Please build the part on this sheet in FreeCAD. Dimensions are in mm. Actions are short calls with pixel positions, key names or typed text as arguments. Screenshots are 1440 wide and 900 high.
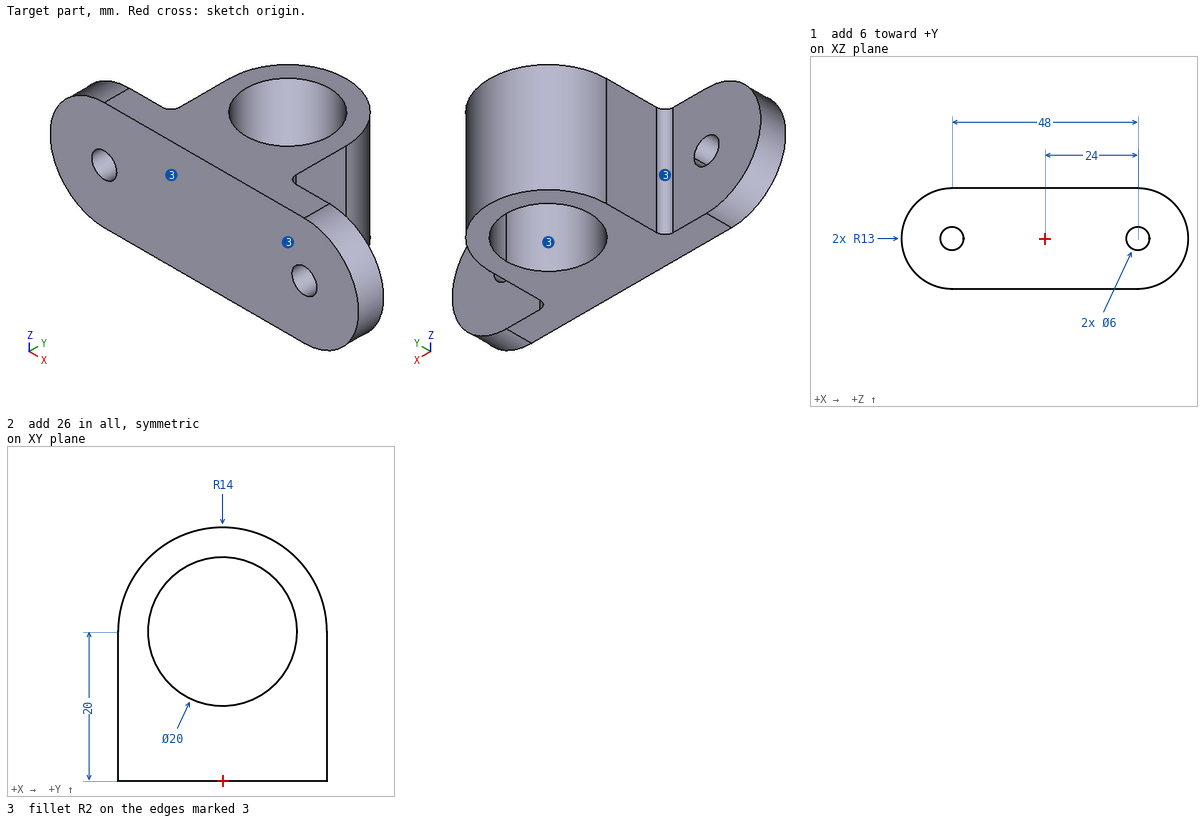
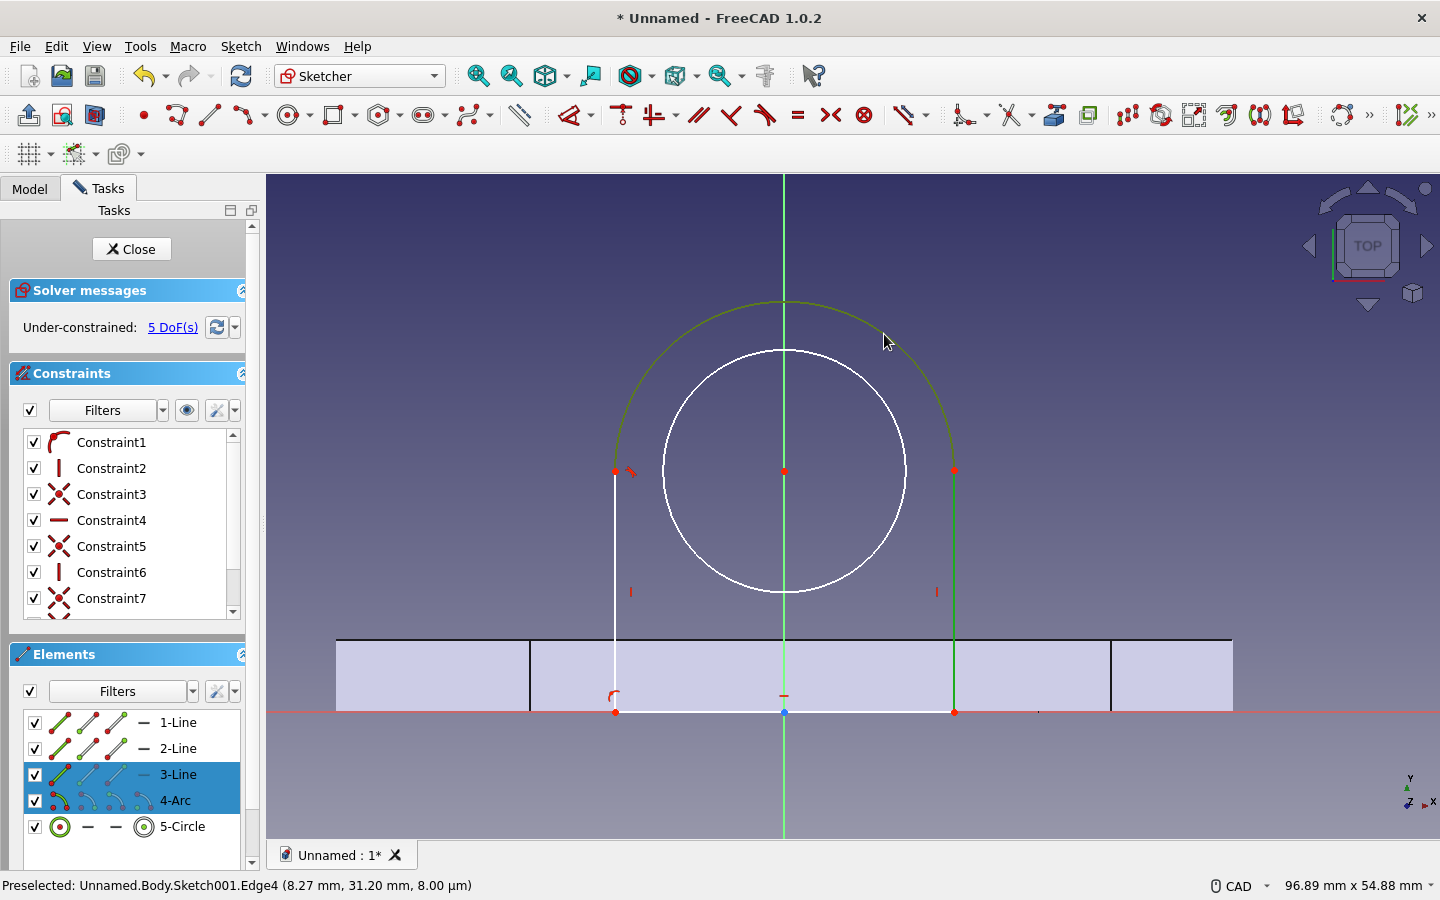
key(t)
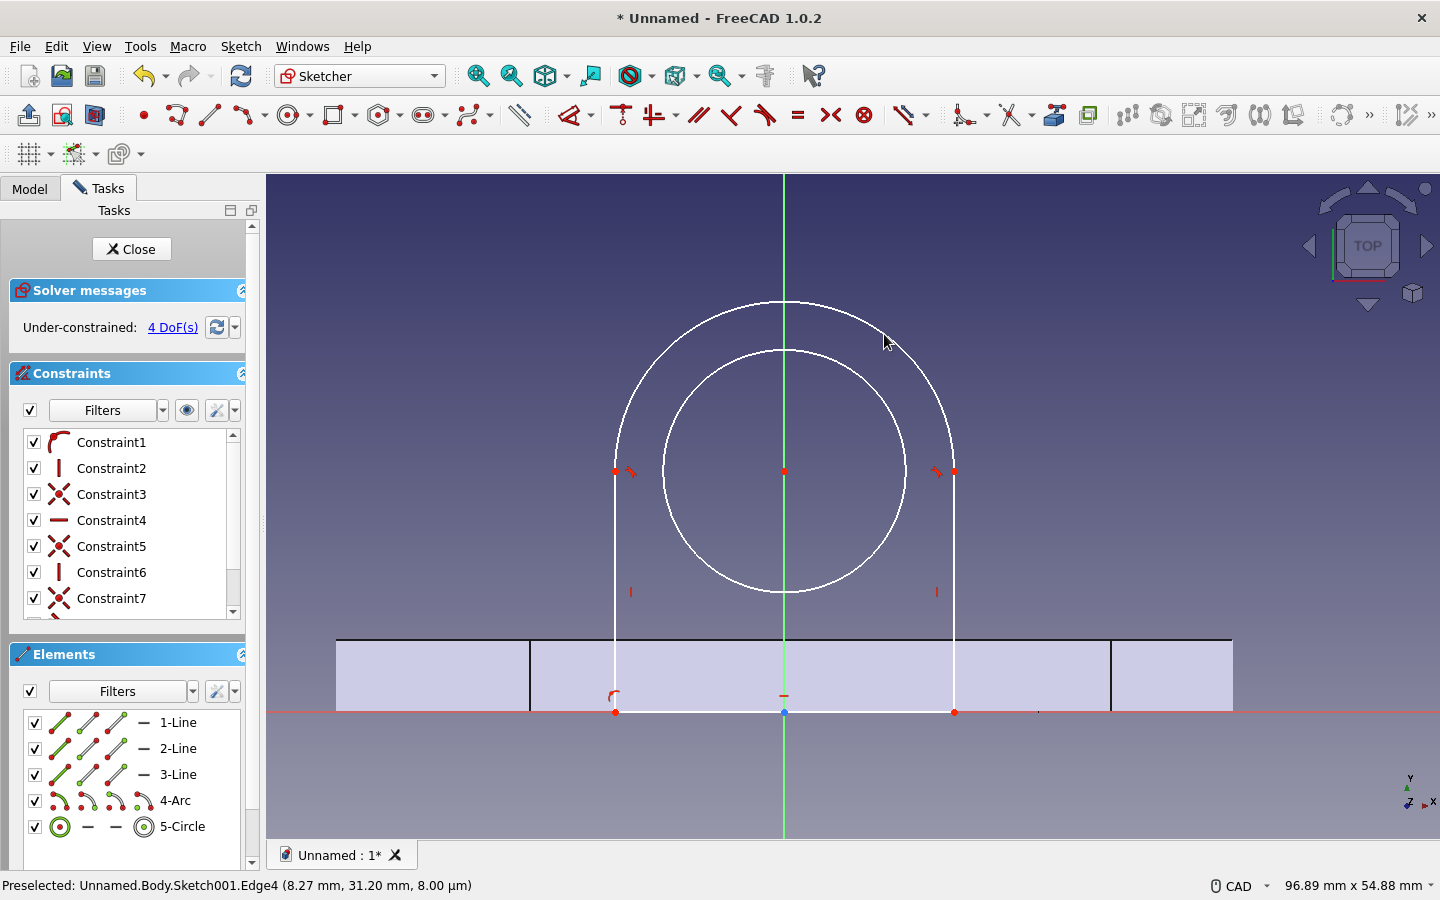
click(784, 471)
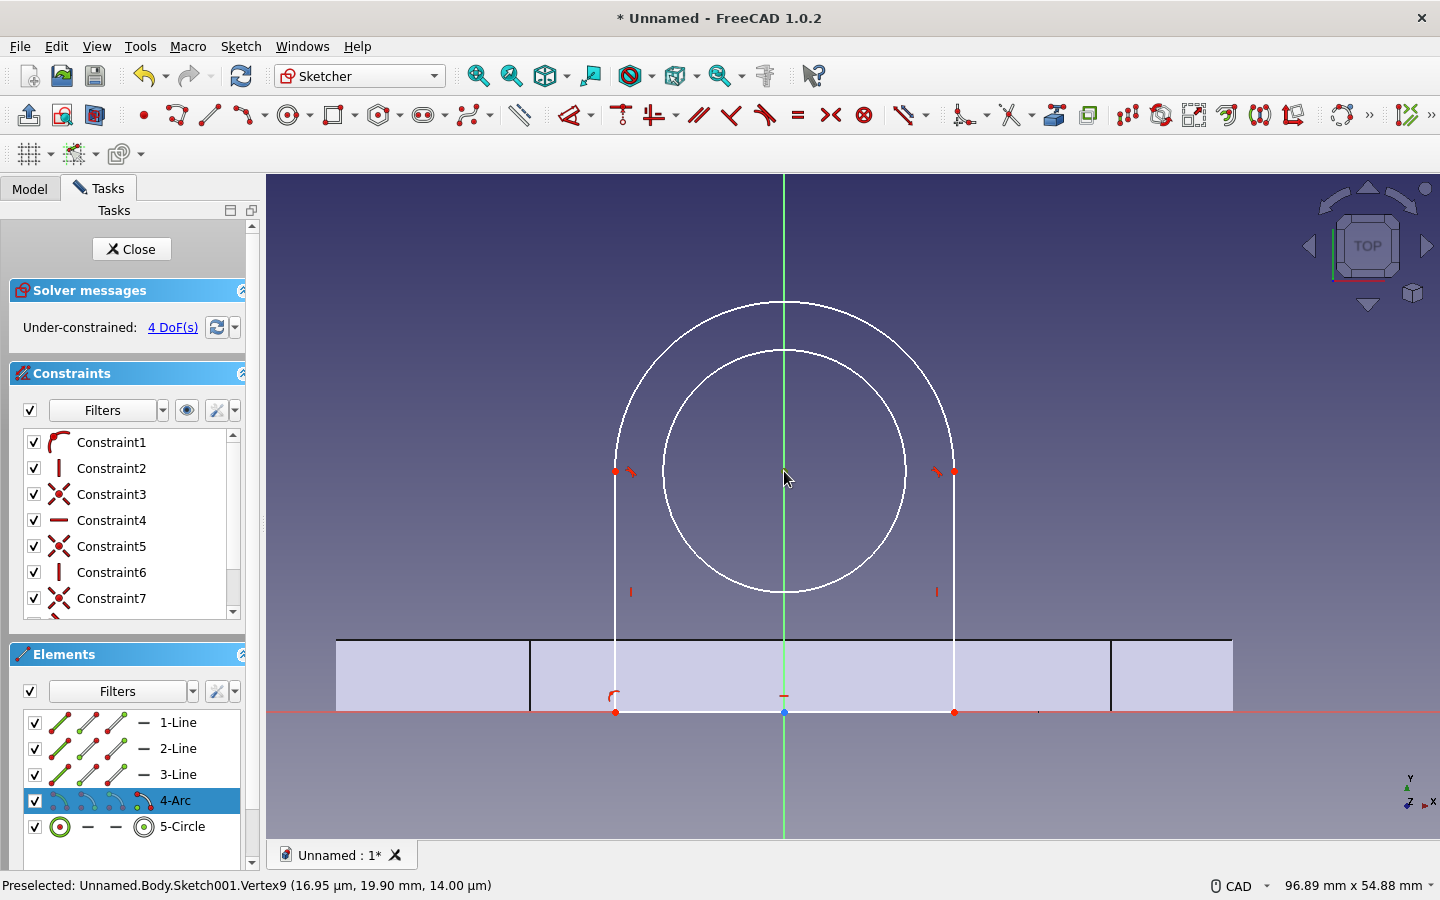
click(784, 768)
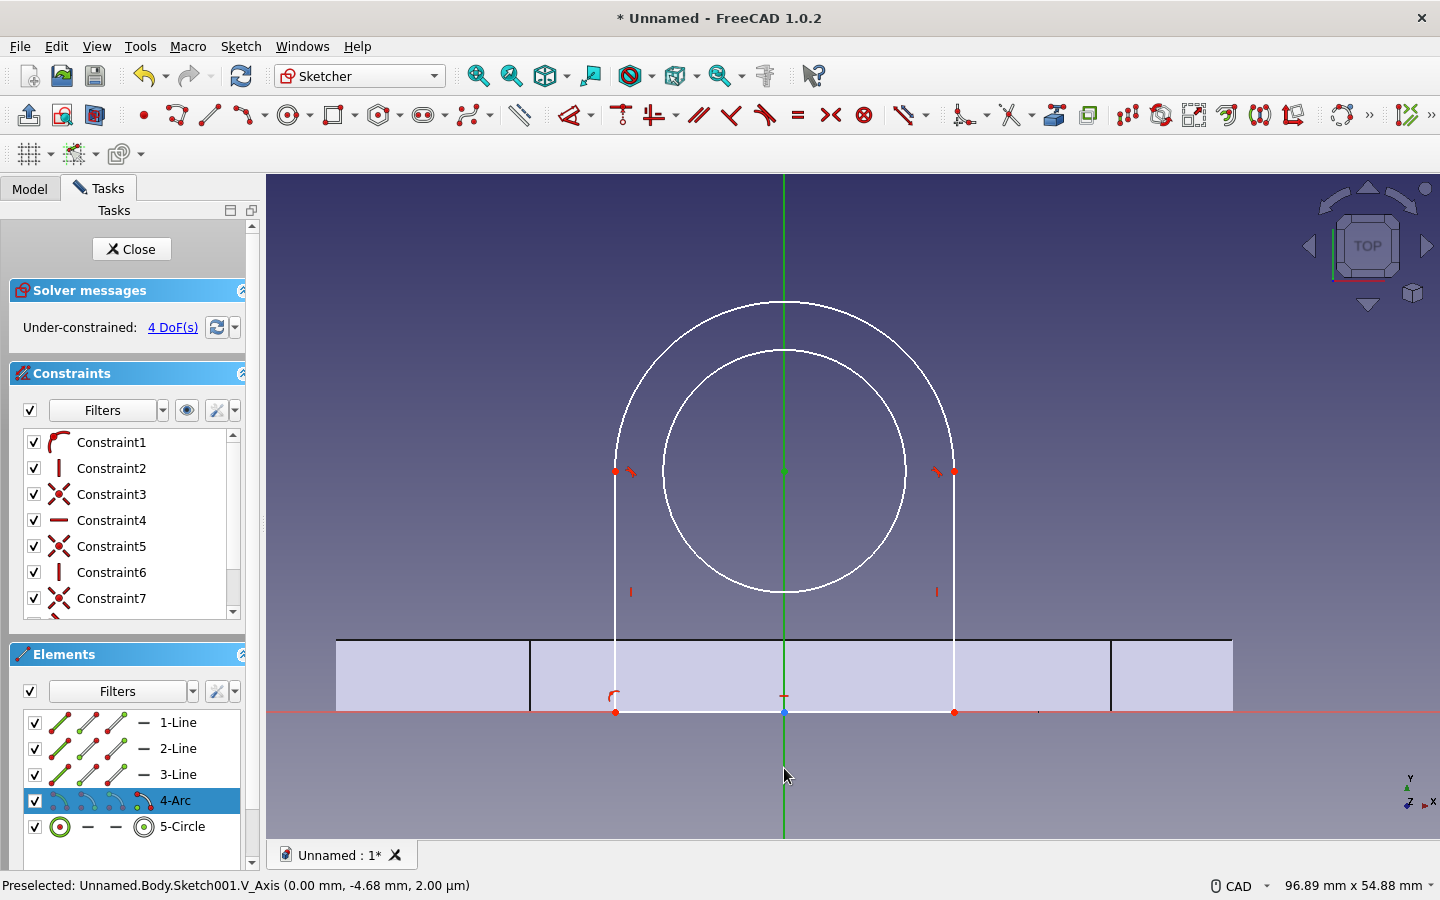
key(c)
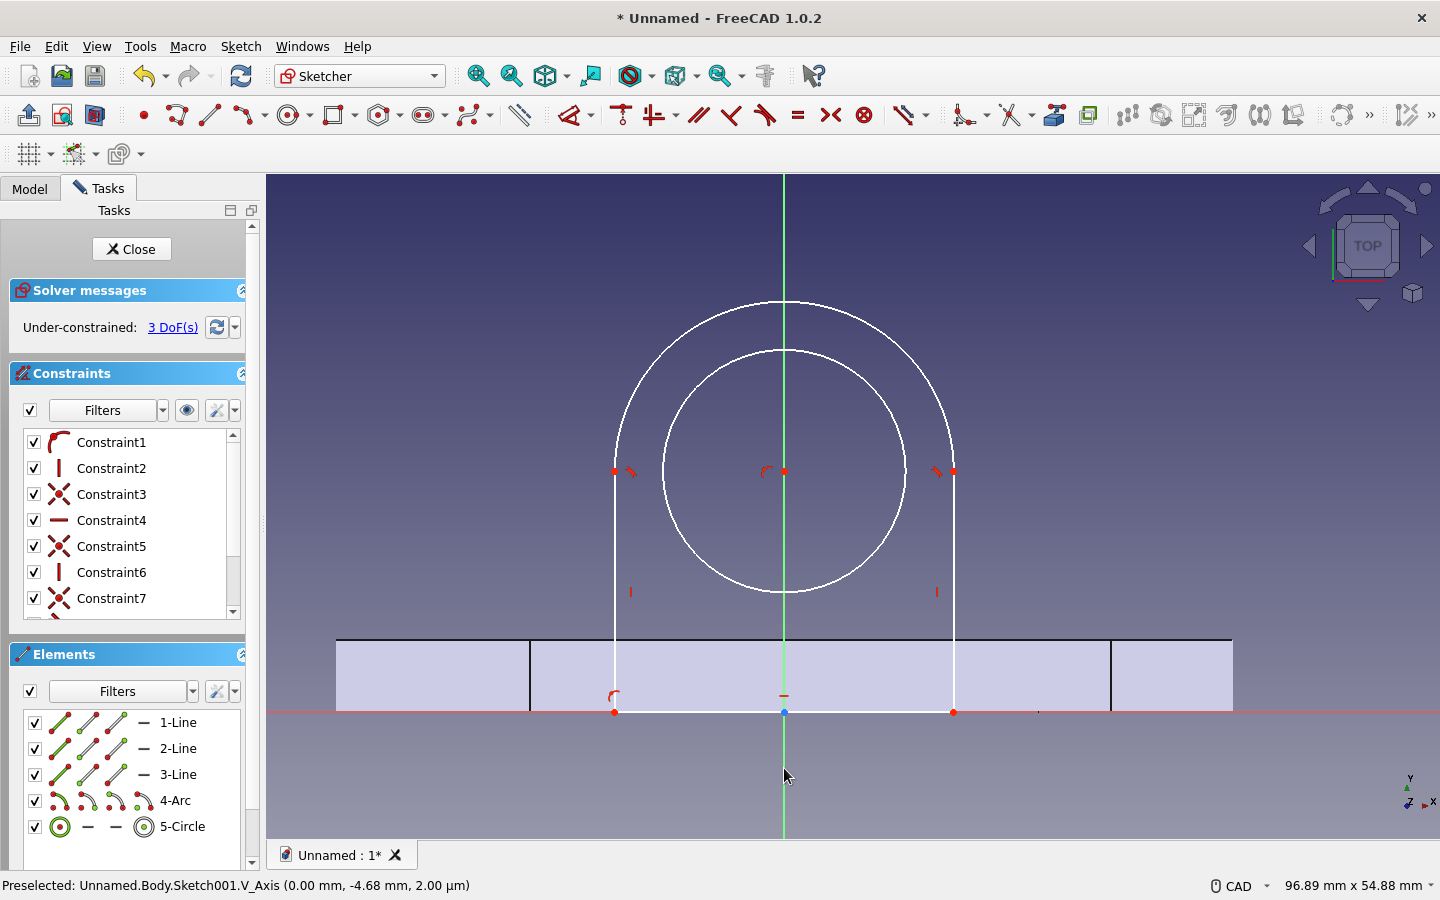
click(884, 334)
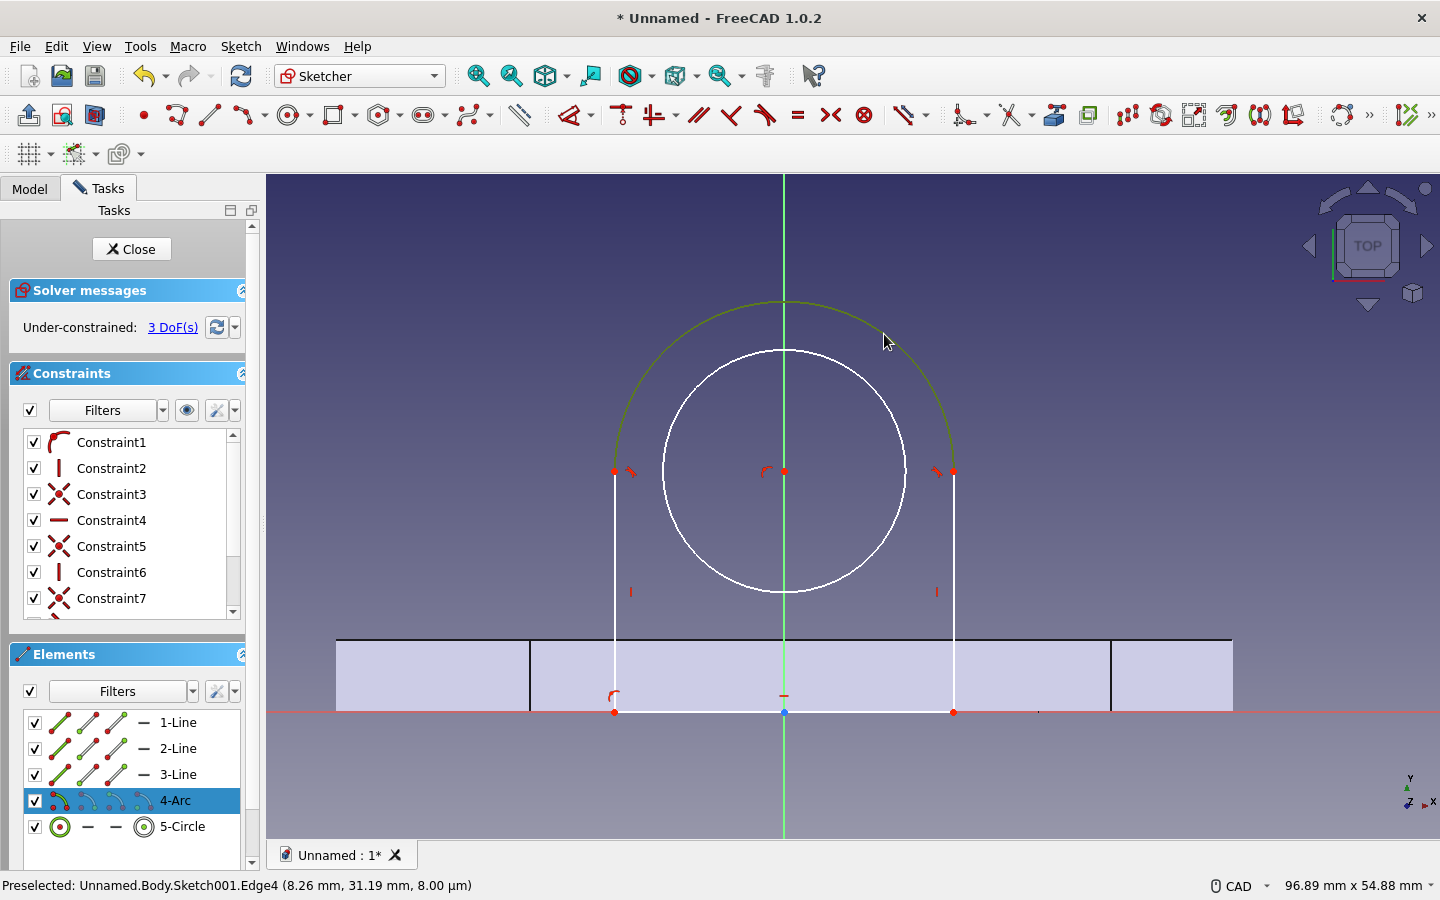
key(k)
key(r)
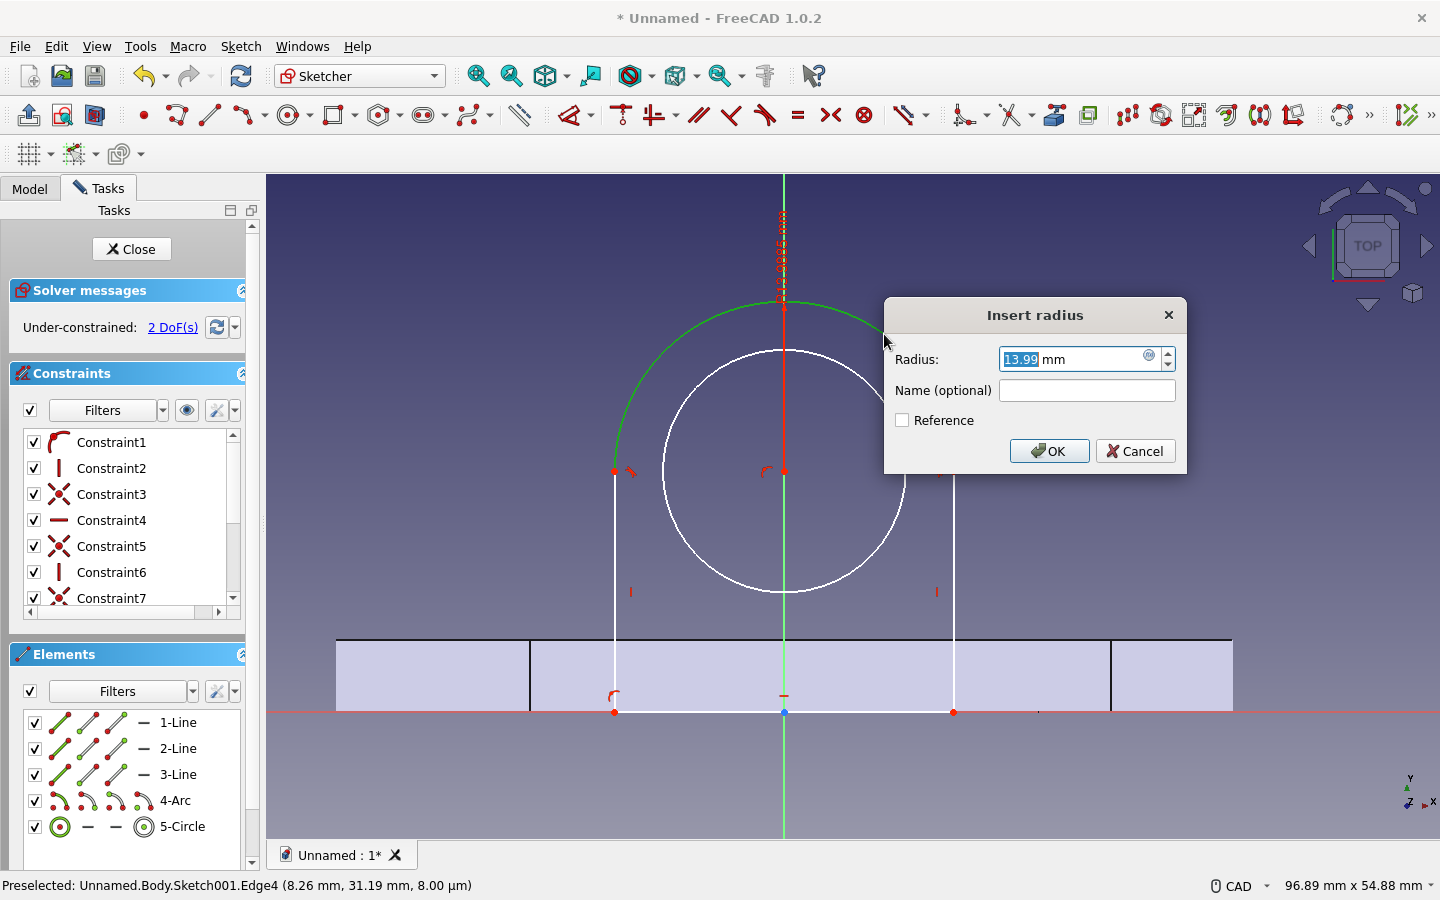
text(14)
key(Return)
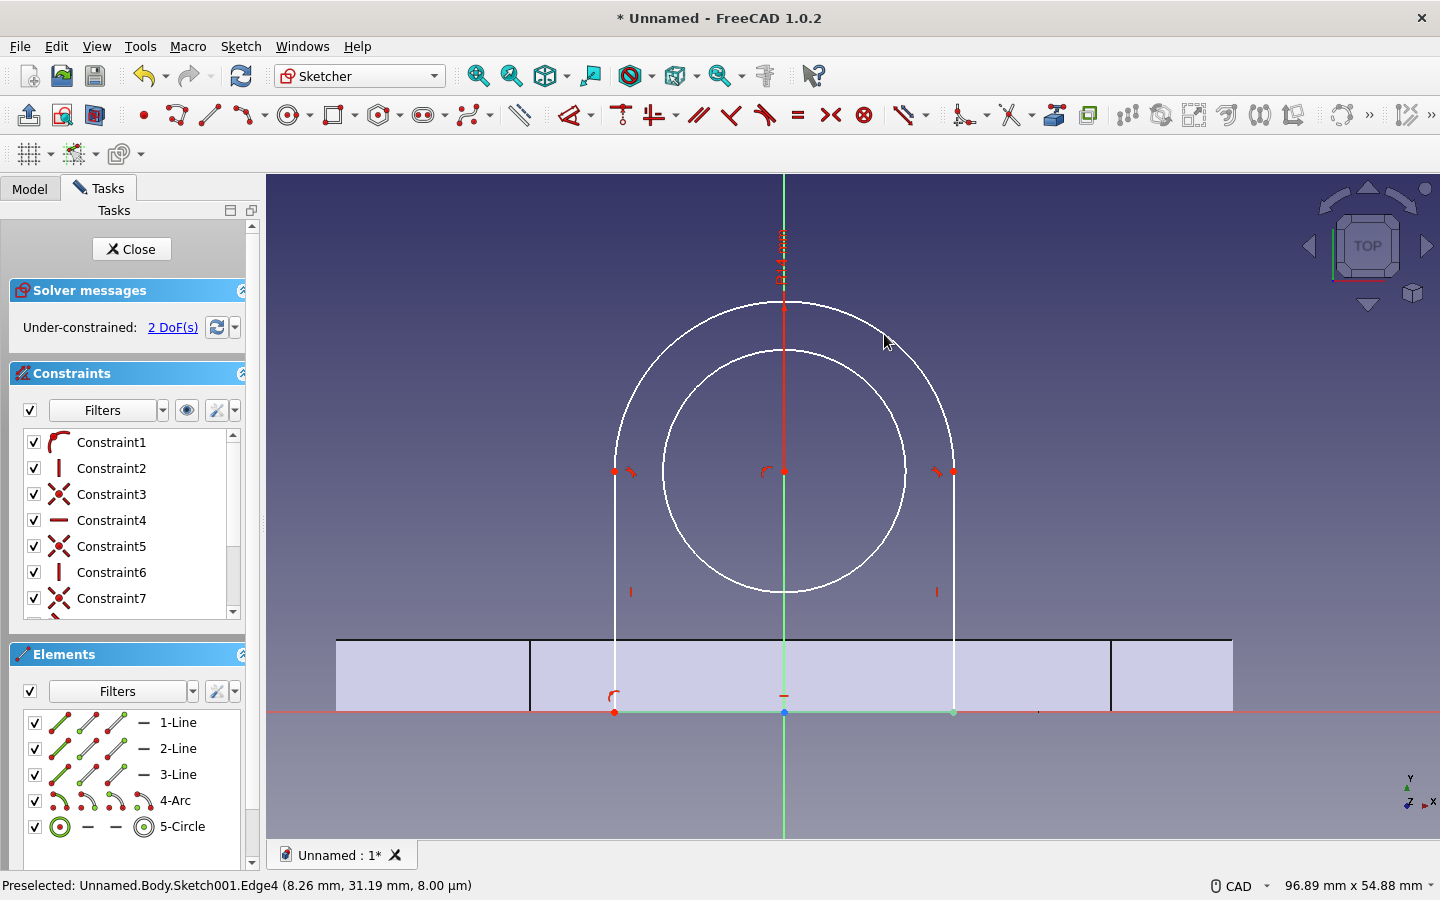
click(870, 385)